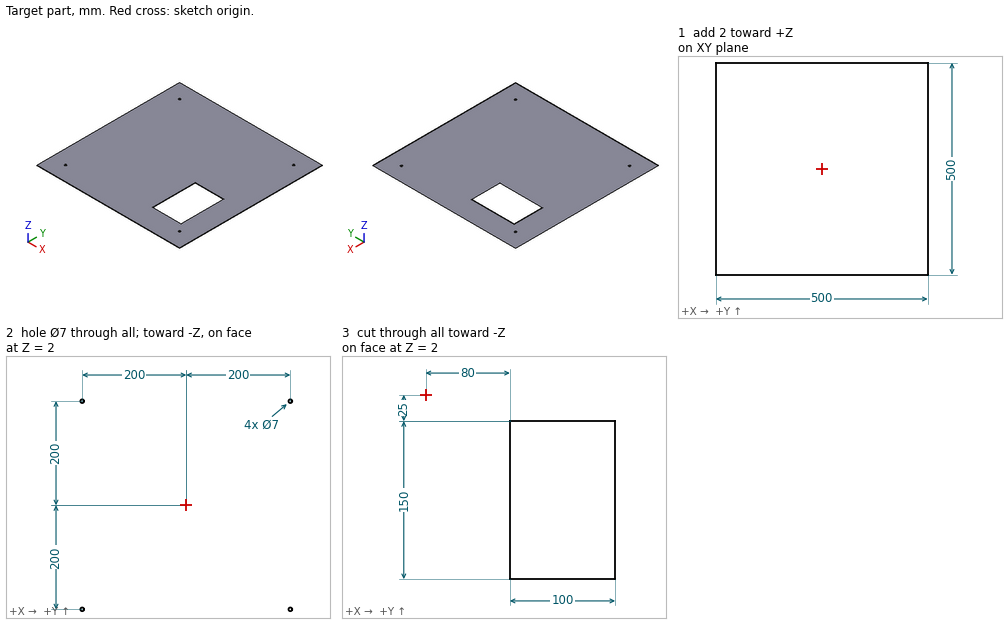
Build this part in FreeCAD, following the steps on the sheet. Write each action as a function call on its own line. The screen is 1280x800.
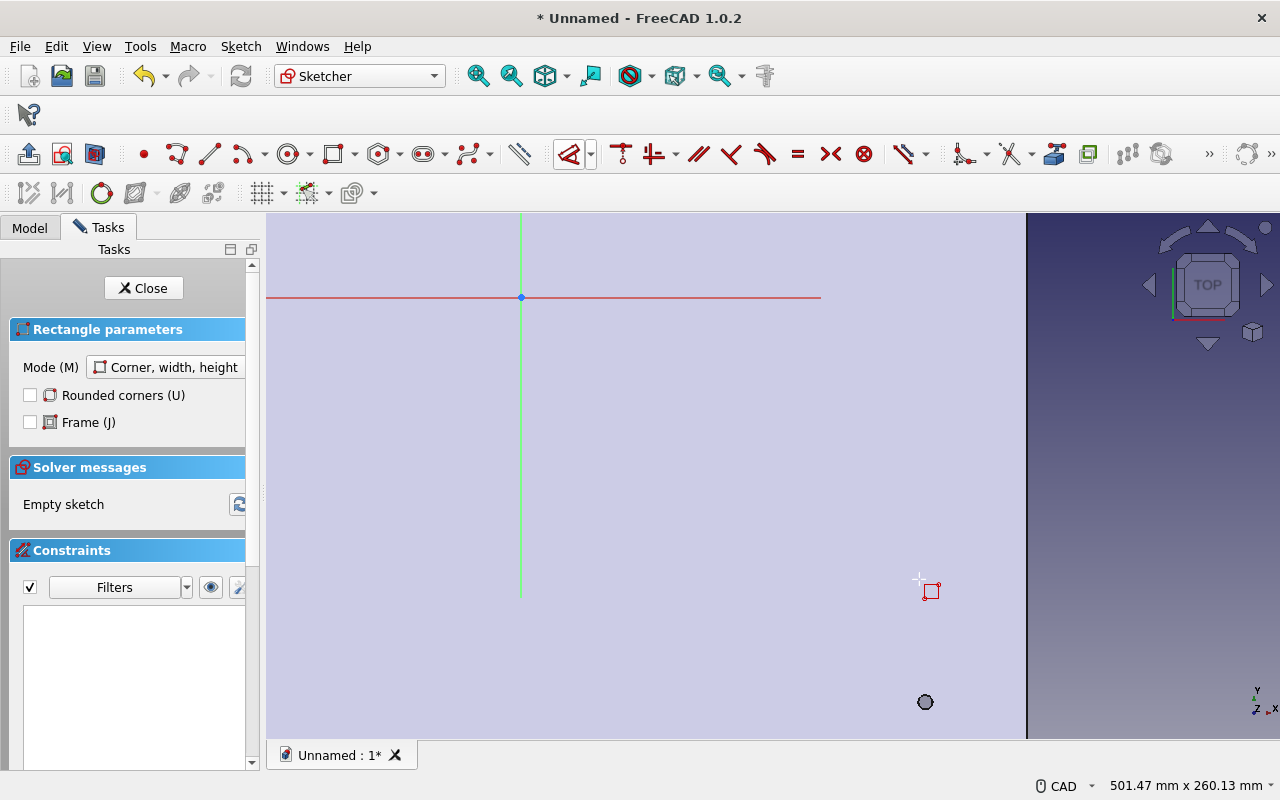
click(683, 348)
click(885, 652)
key(Escape)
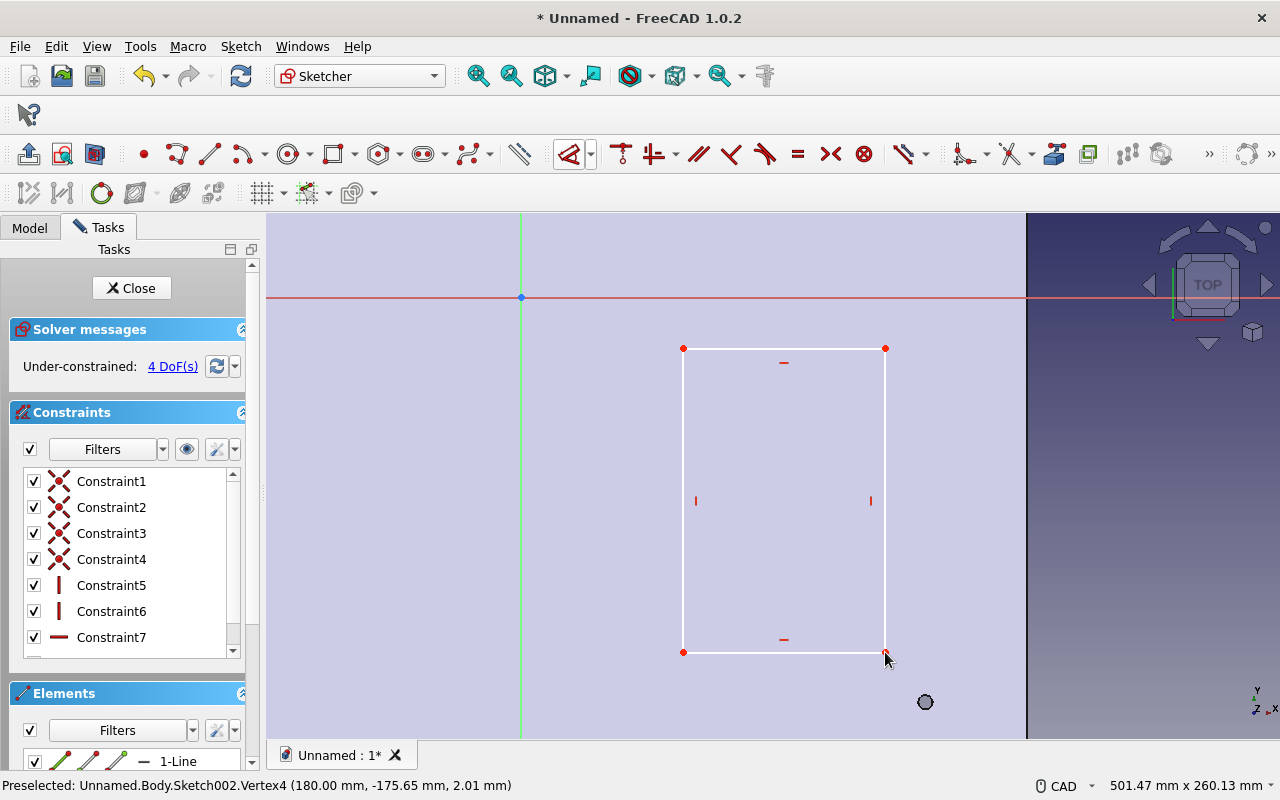
click(683, 440)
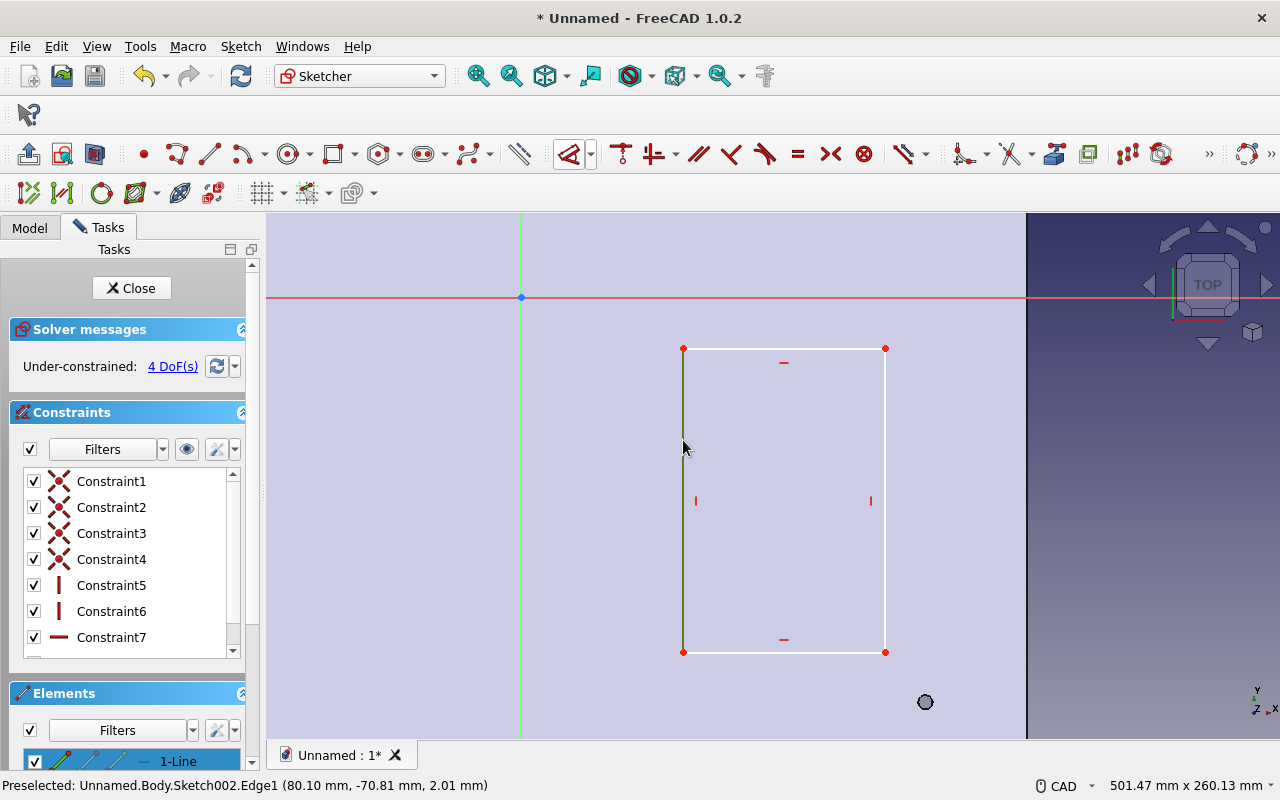
key(i)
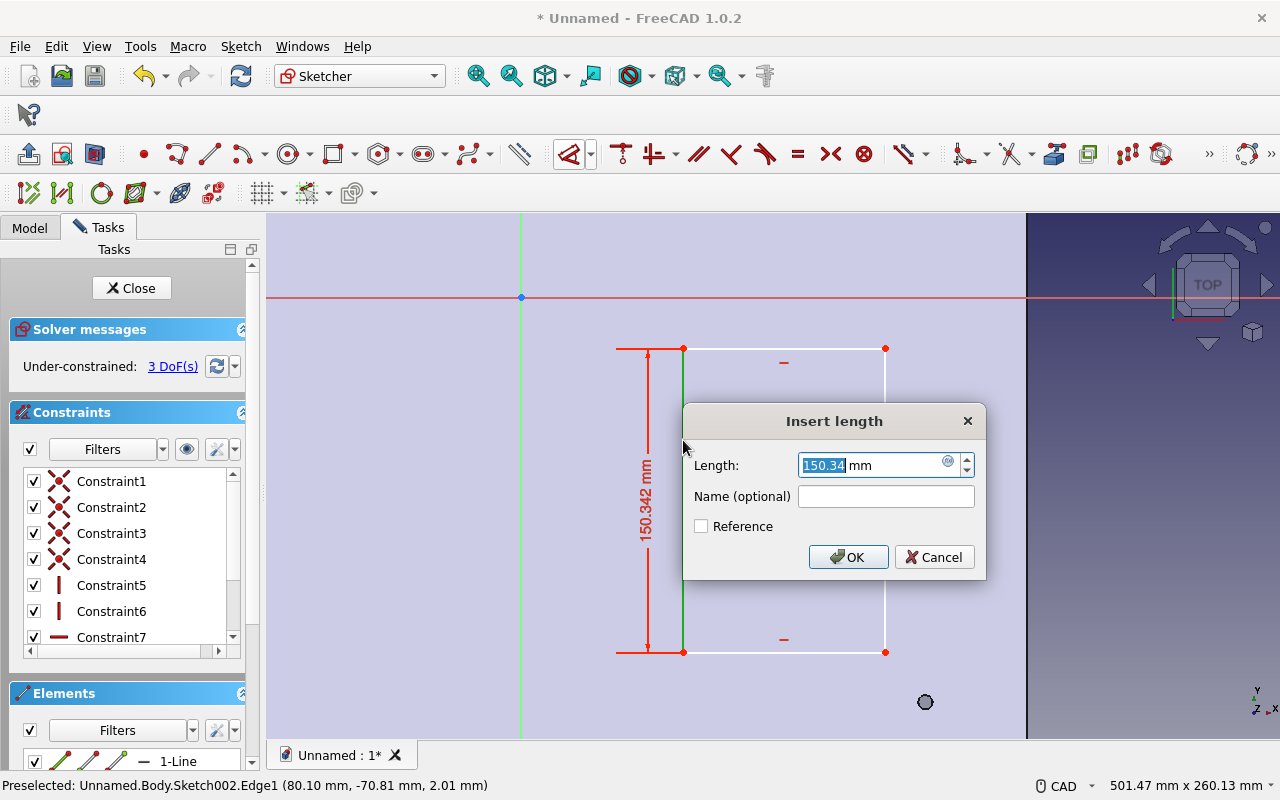
text(150)
key(Return)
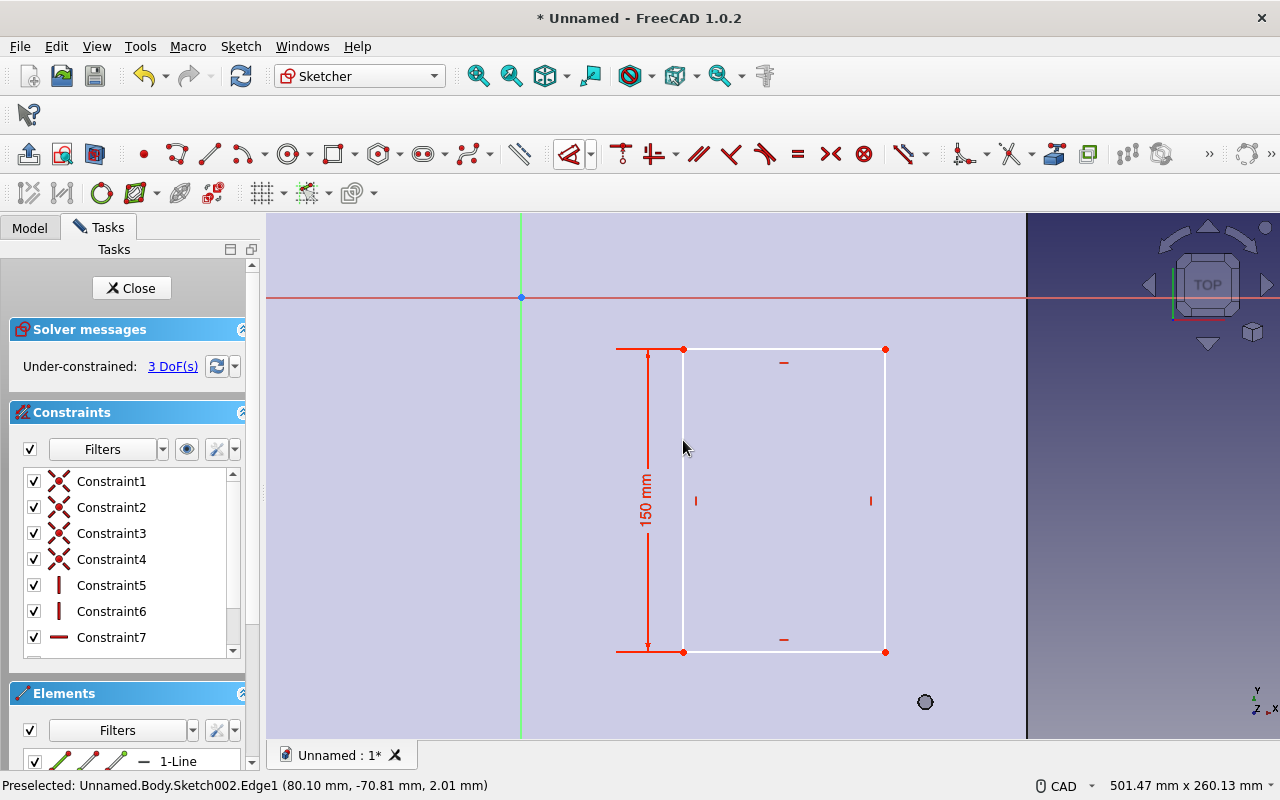
click(744, 652)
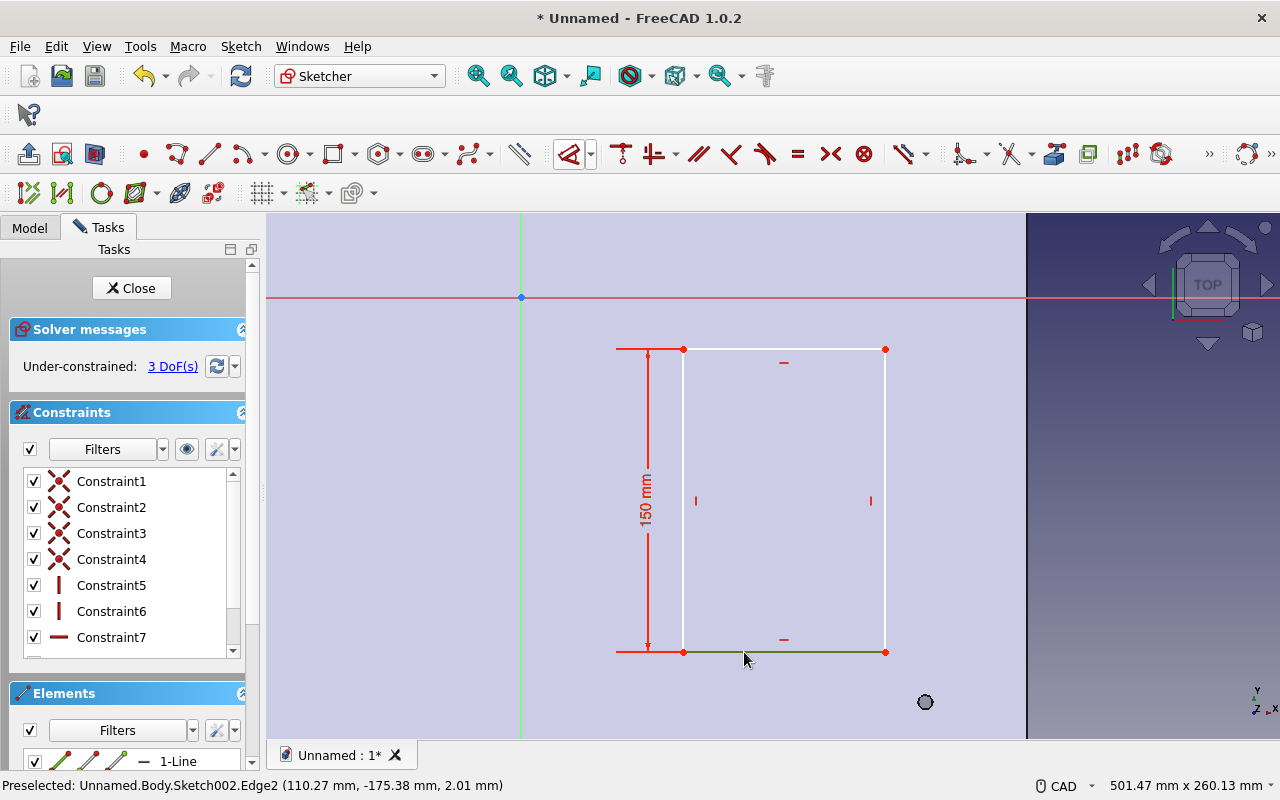
key(l)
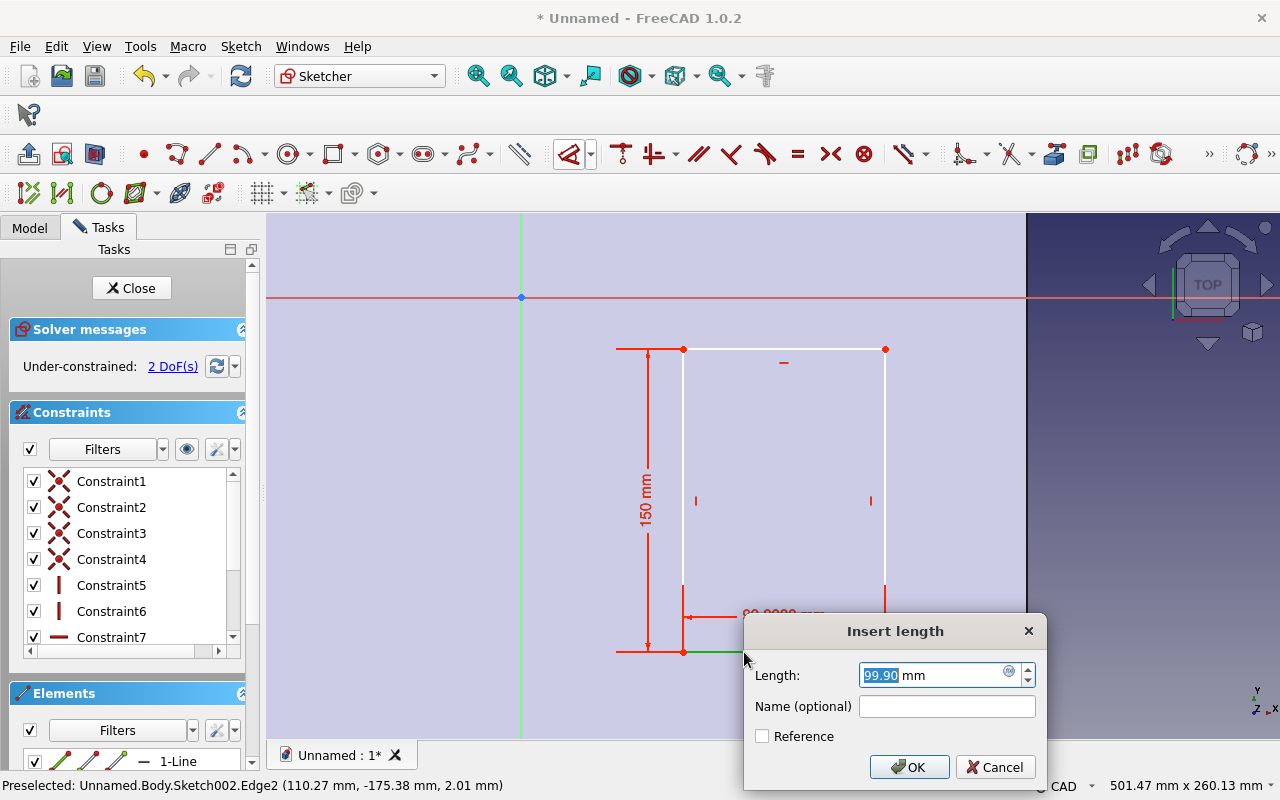
text(100)
key(Return)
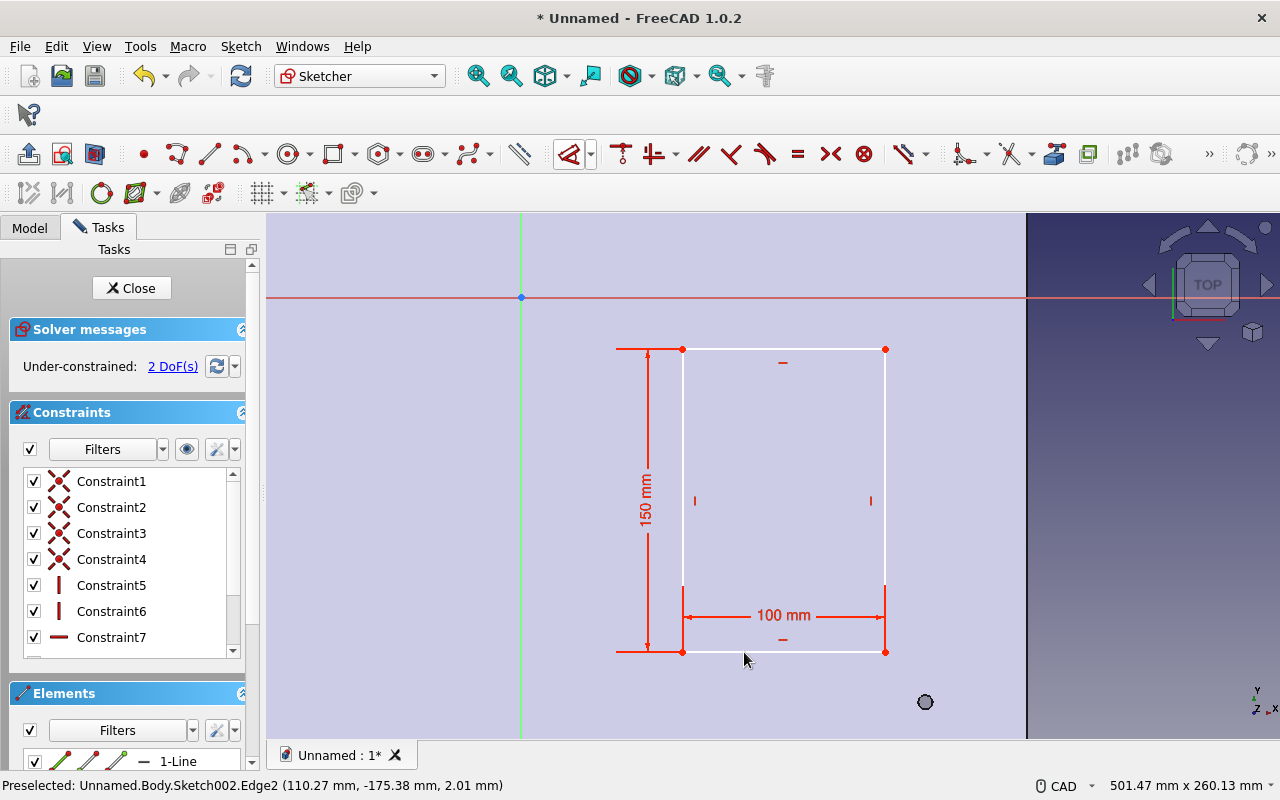
click(683, 349)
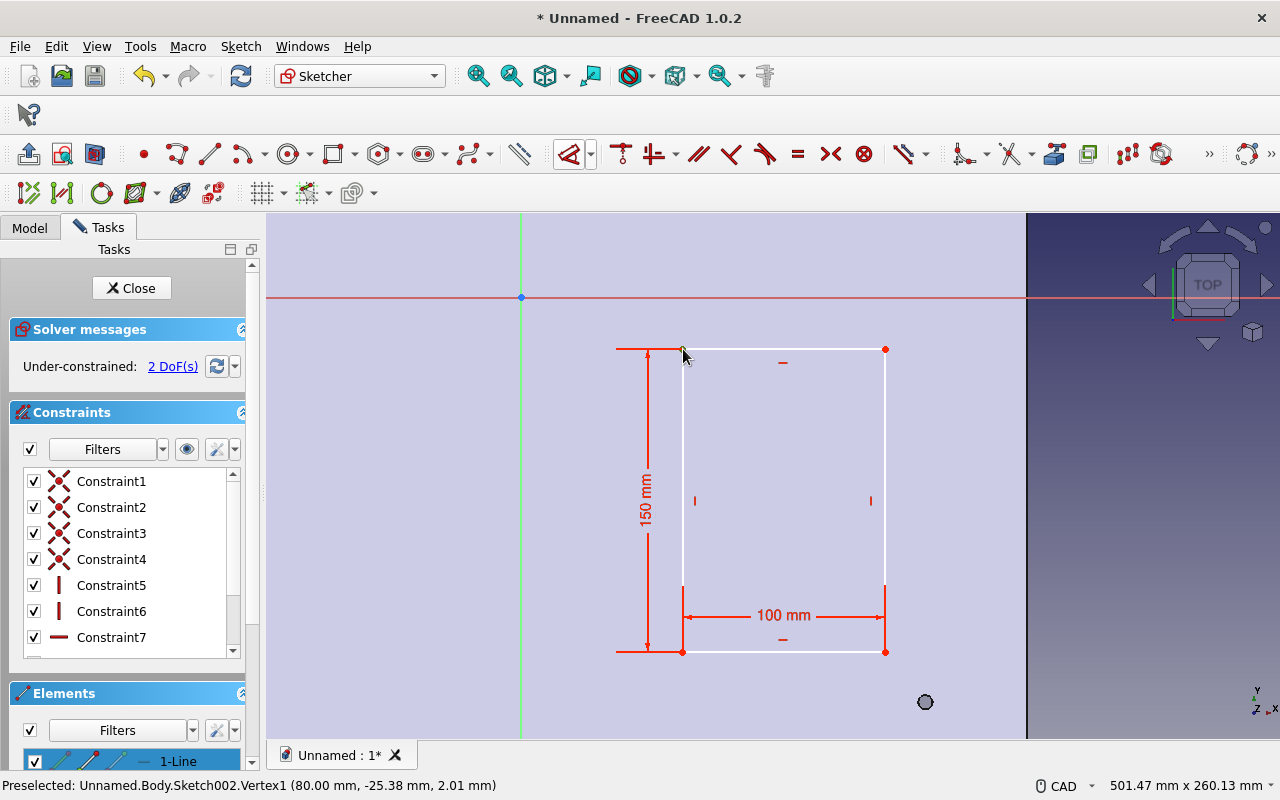
key(l)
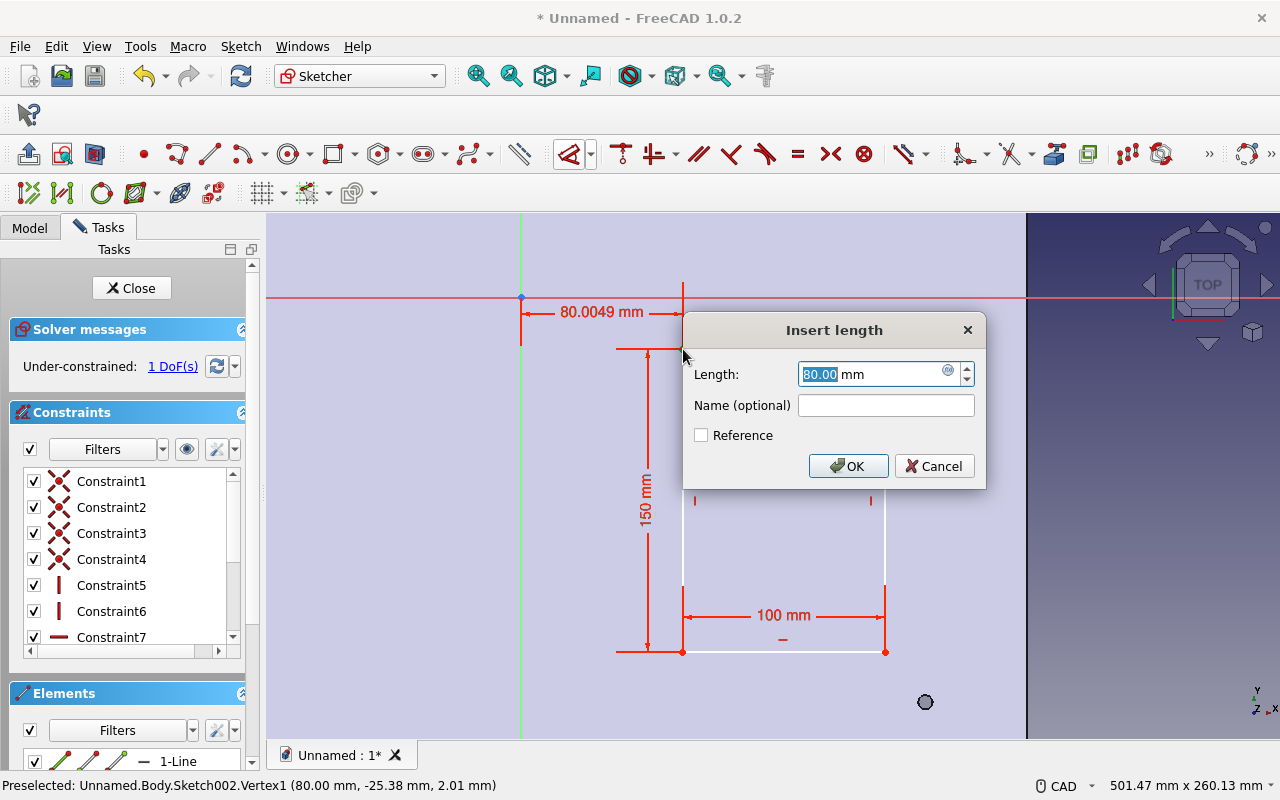
text(80)
key(Return)